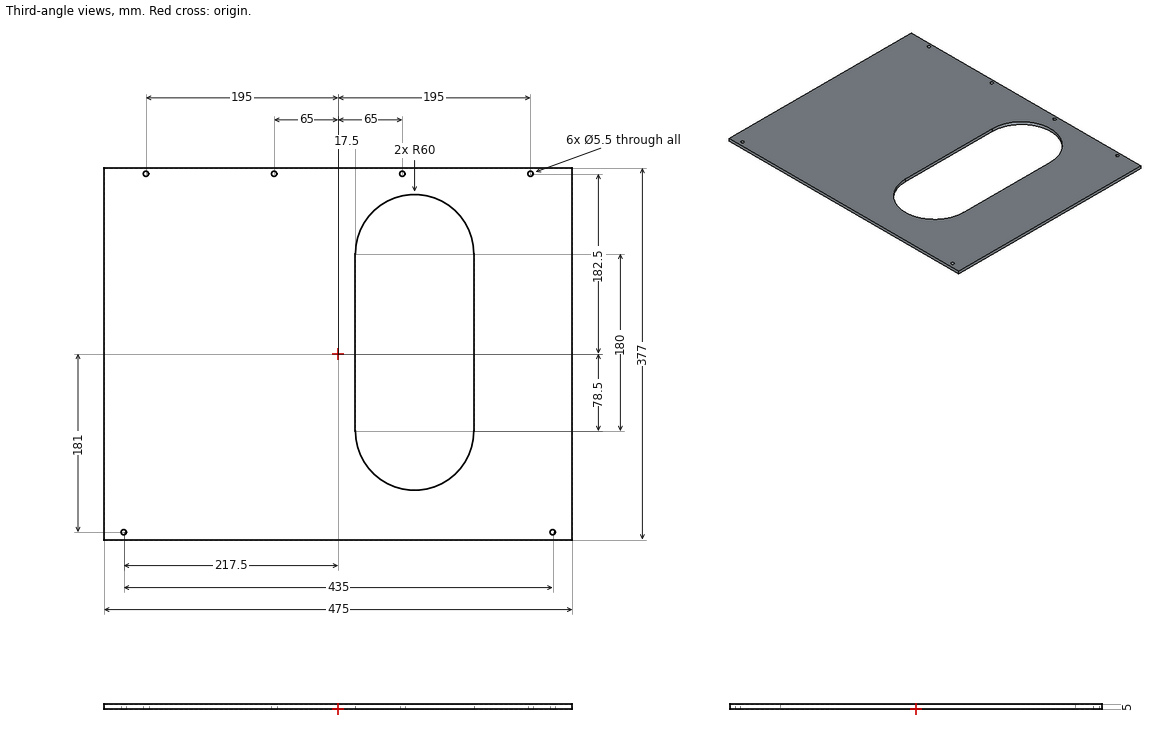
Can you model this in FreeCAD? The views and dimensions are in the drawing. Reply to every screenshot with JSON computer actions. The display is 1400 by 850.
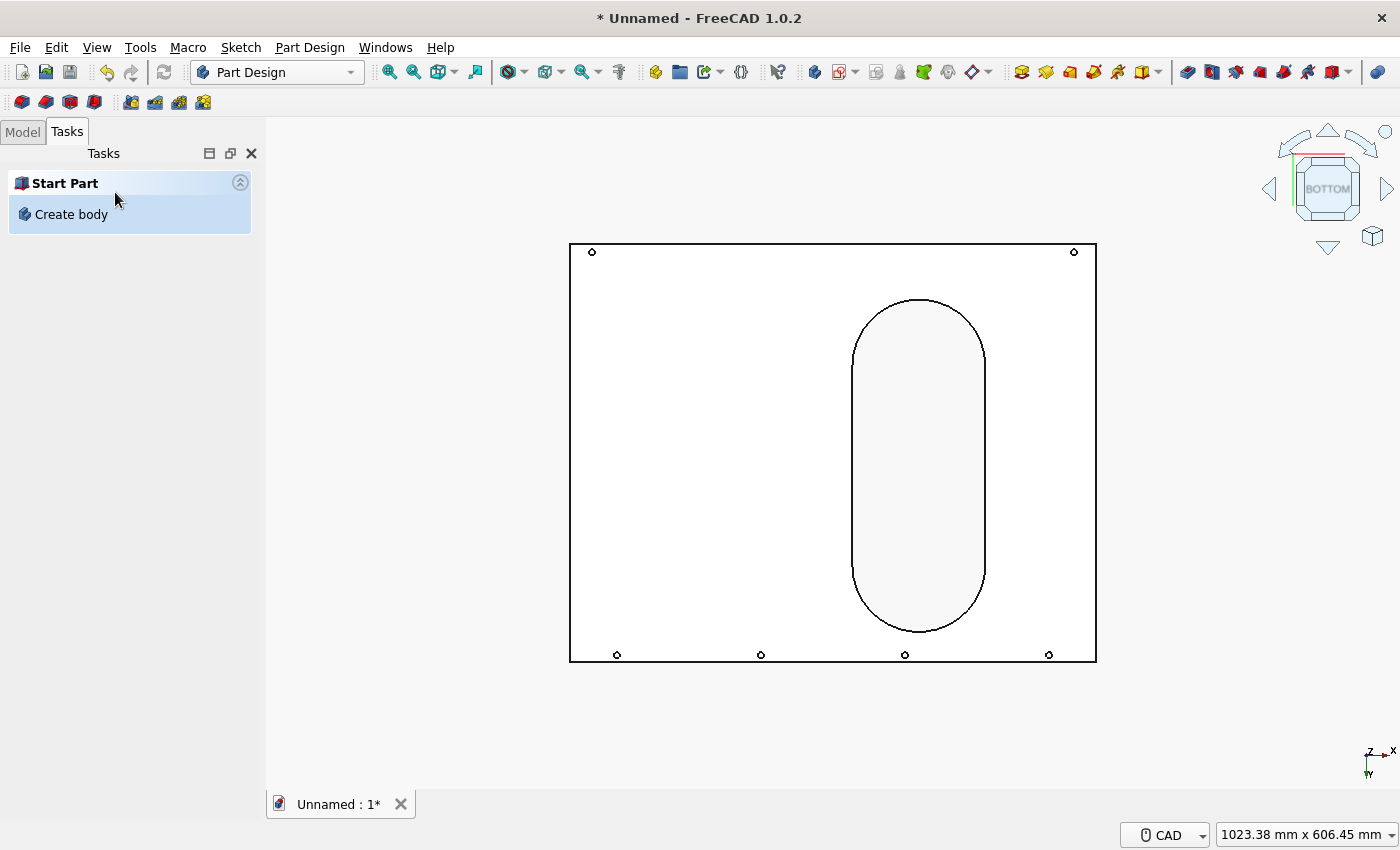
{"action": "key", "text": "0"}